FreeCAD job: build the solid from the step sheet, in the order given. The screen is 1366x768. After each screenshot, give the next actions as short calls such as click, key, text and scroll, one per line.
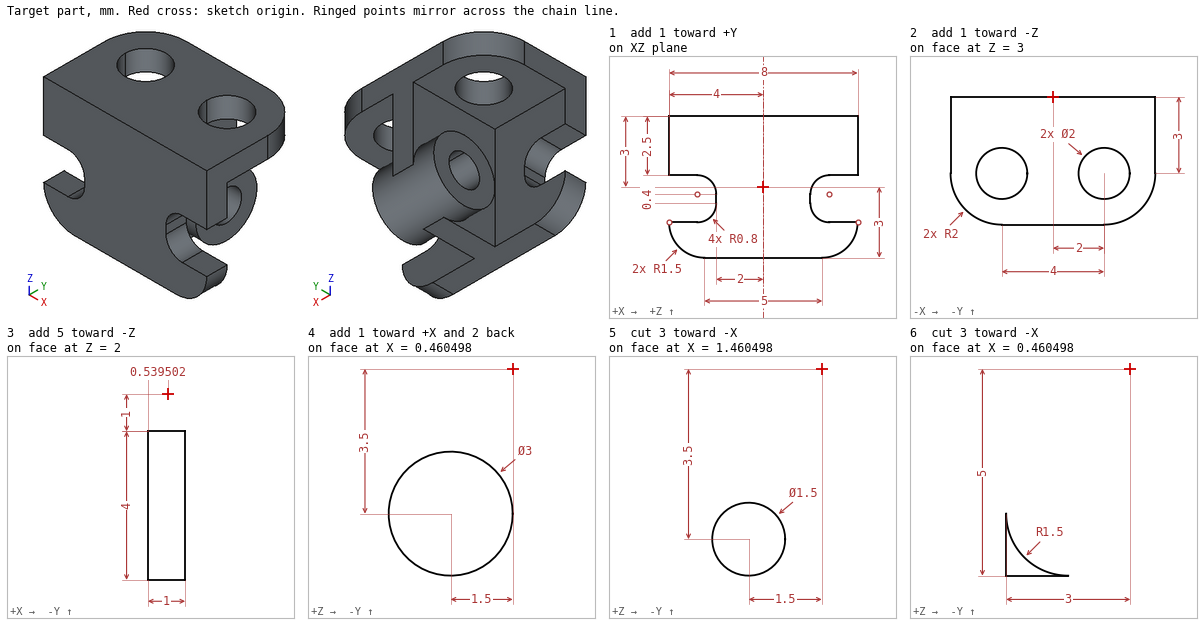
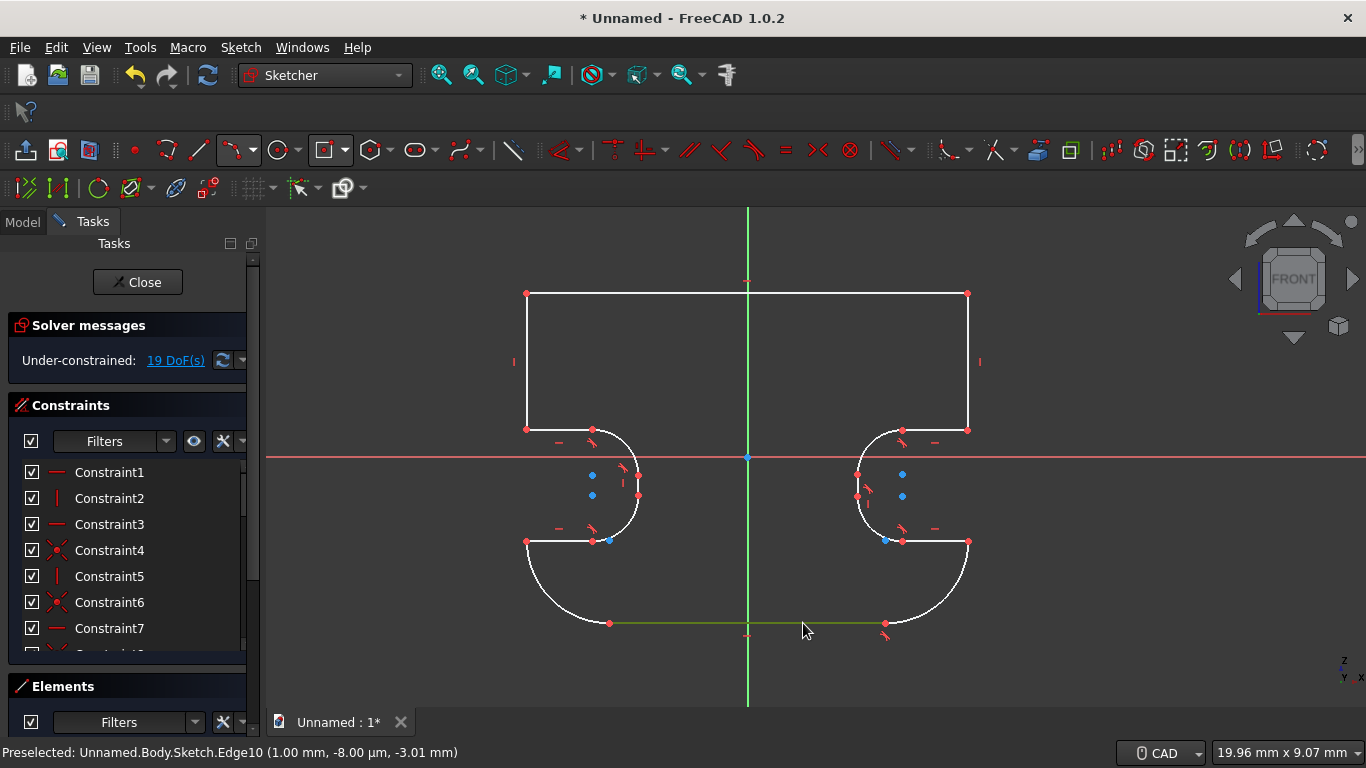
click(536, 579)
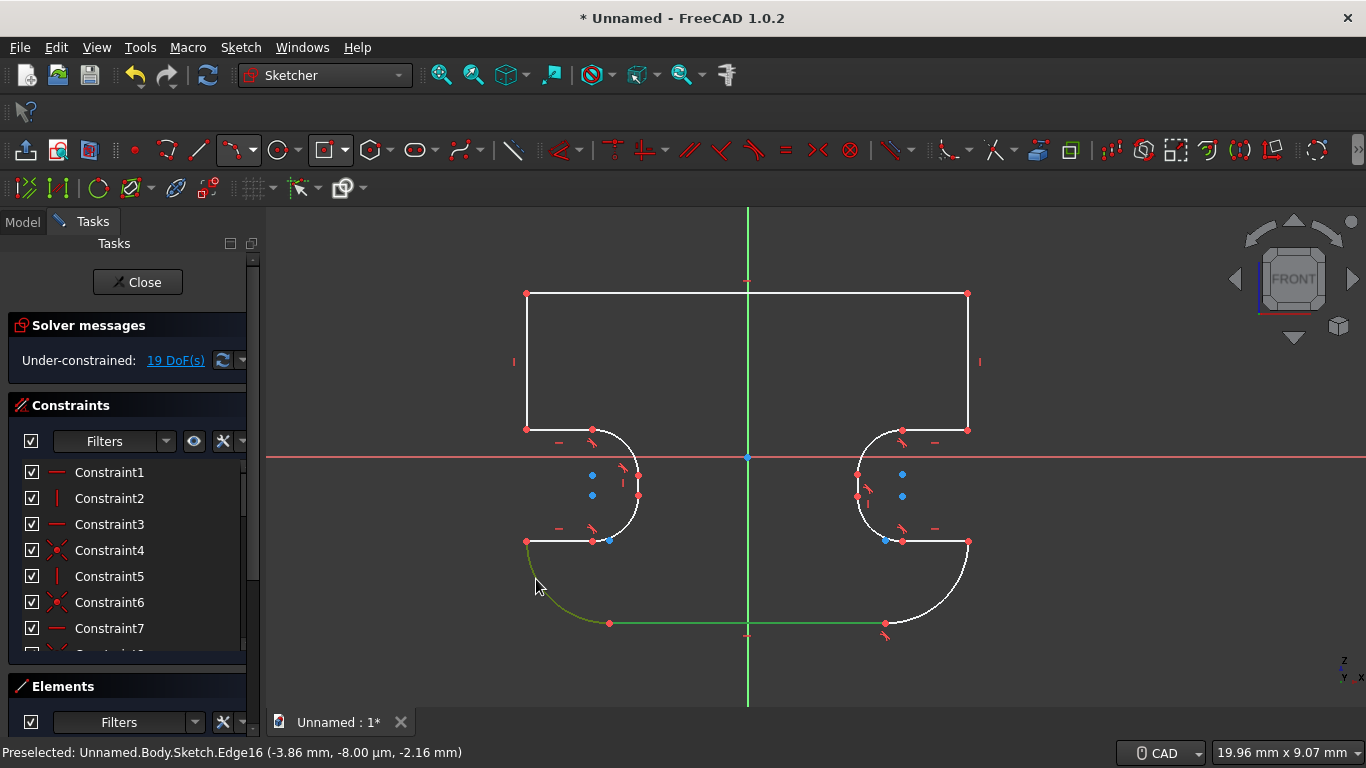
click(754, 150)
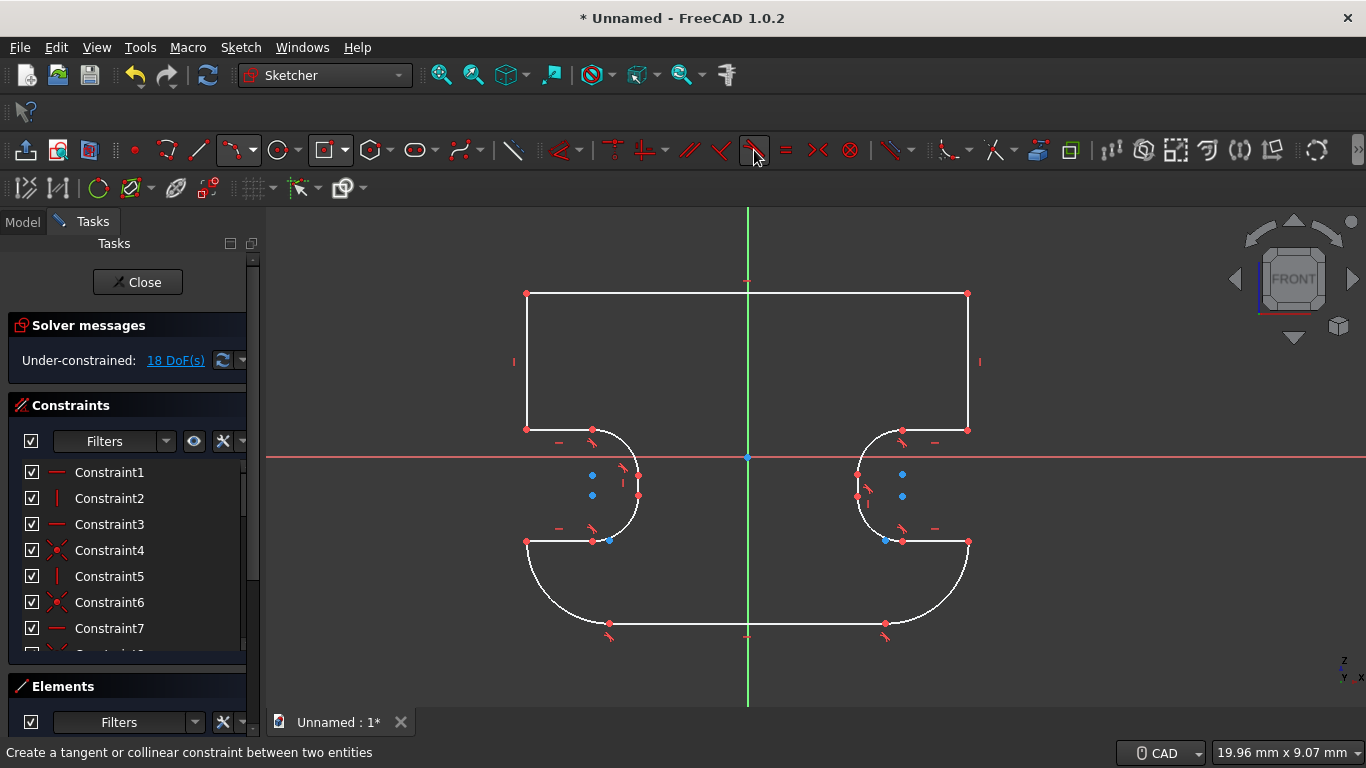
click(633, 516)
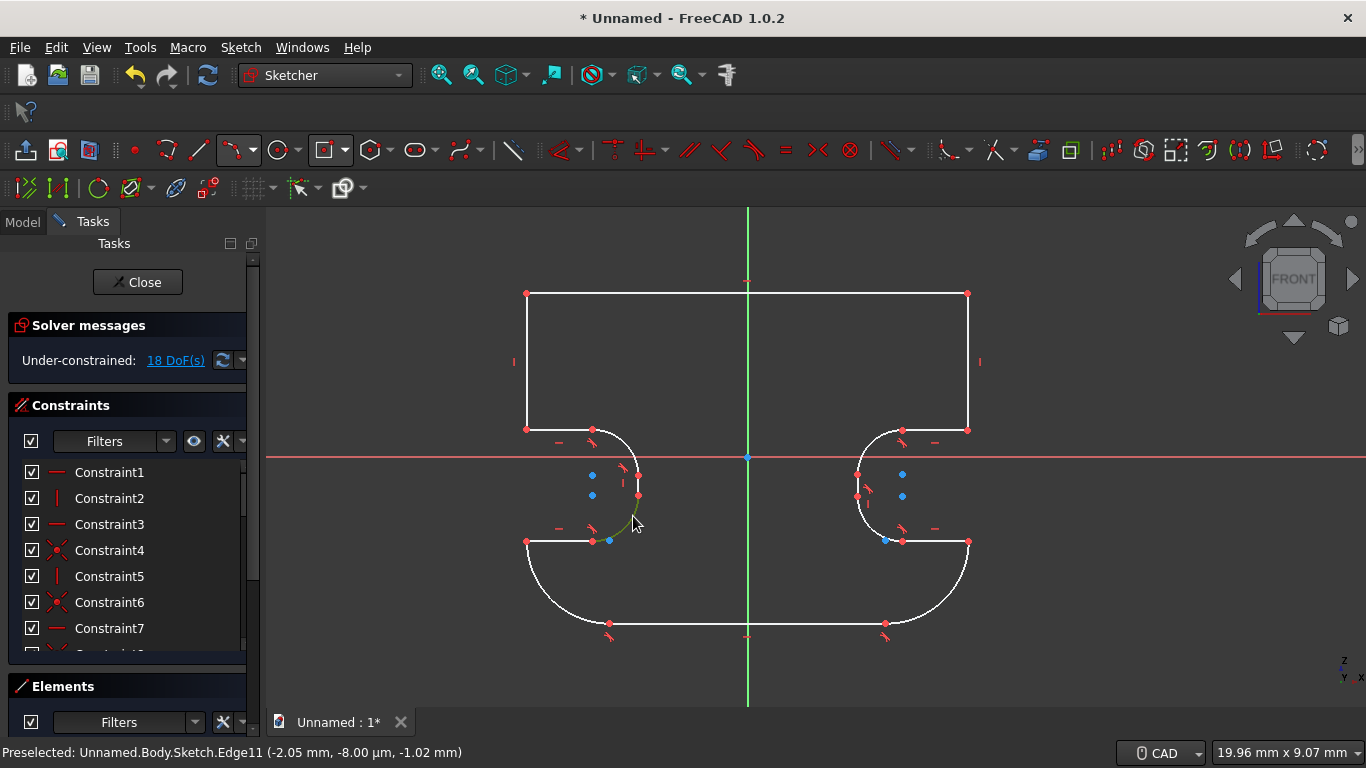
click(633, 455)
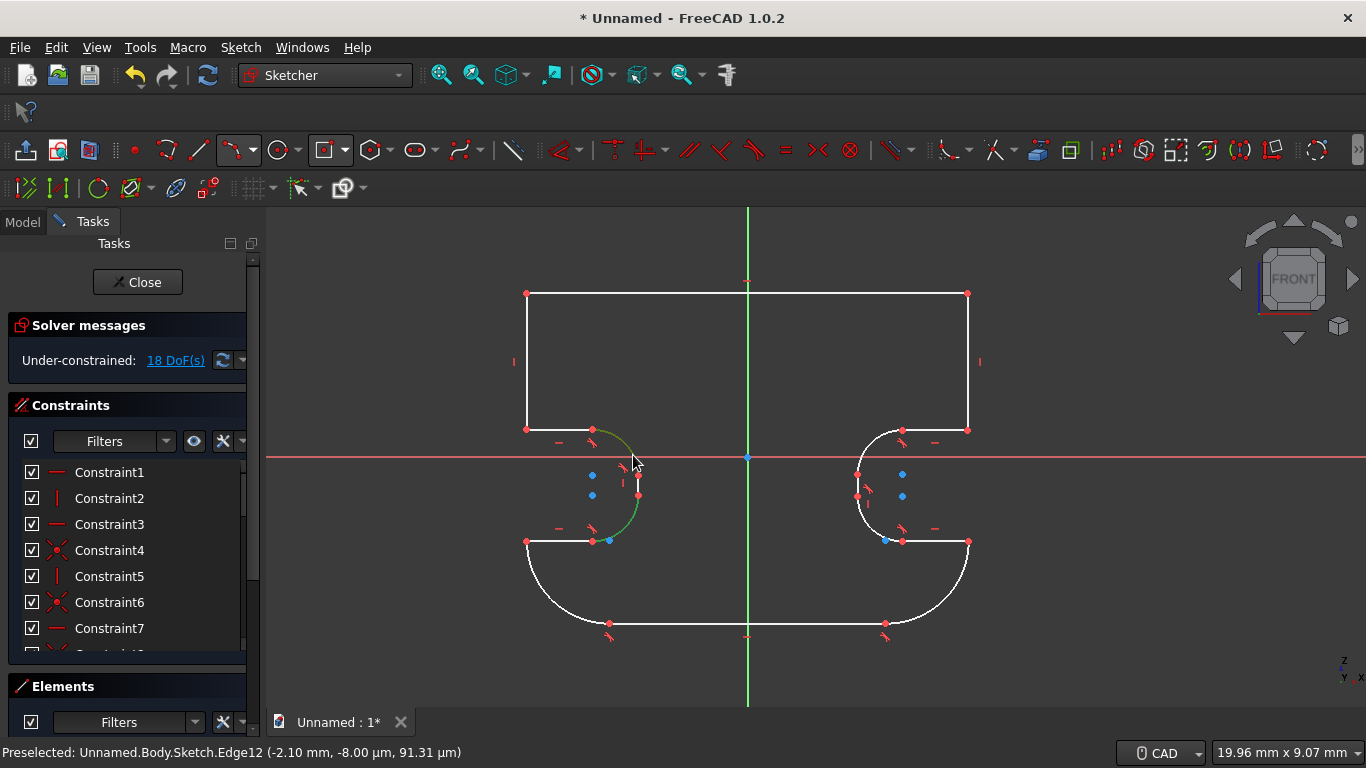
click(882, 435)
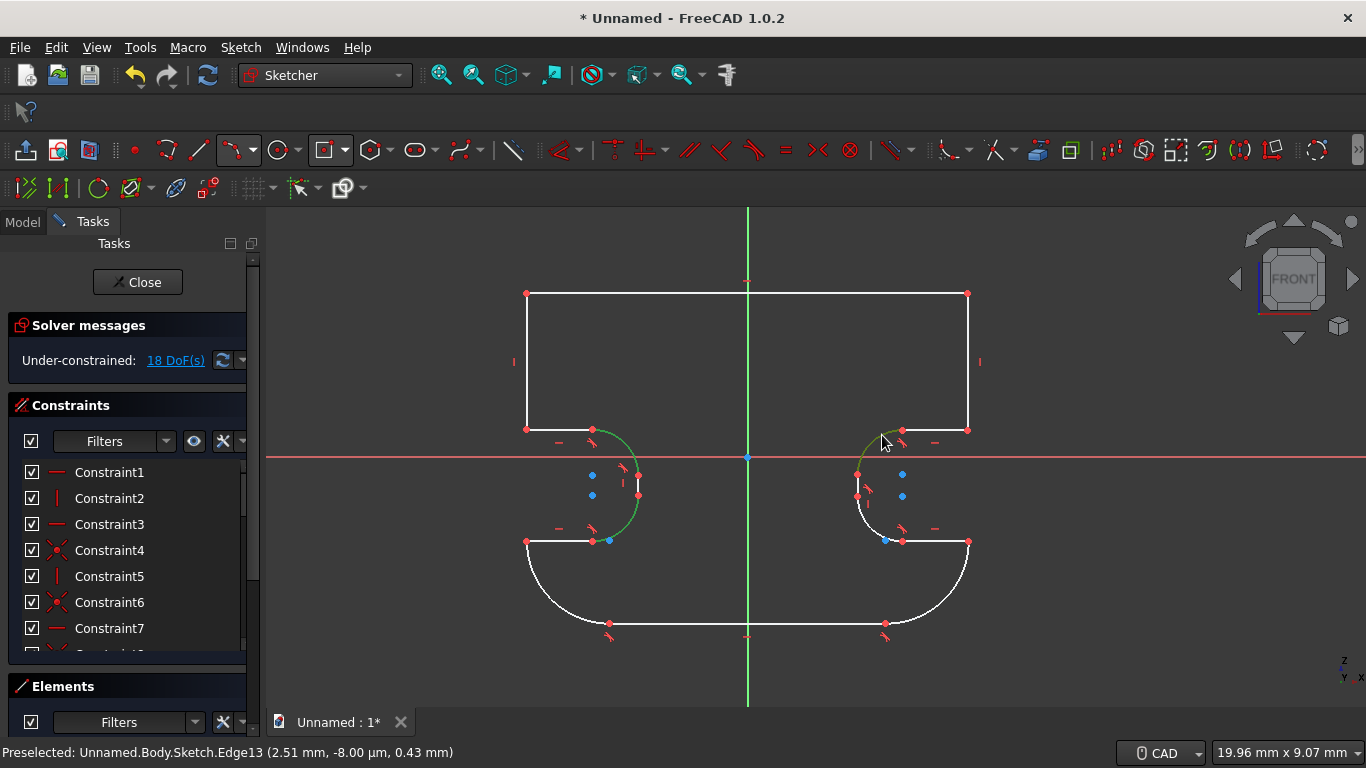
click(863, 517)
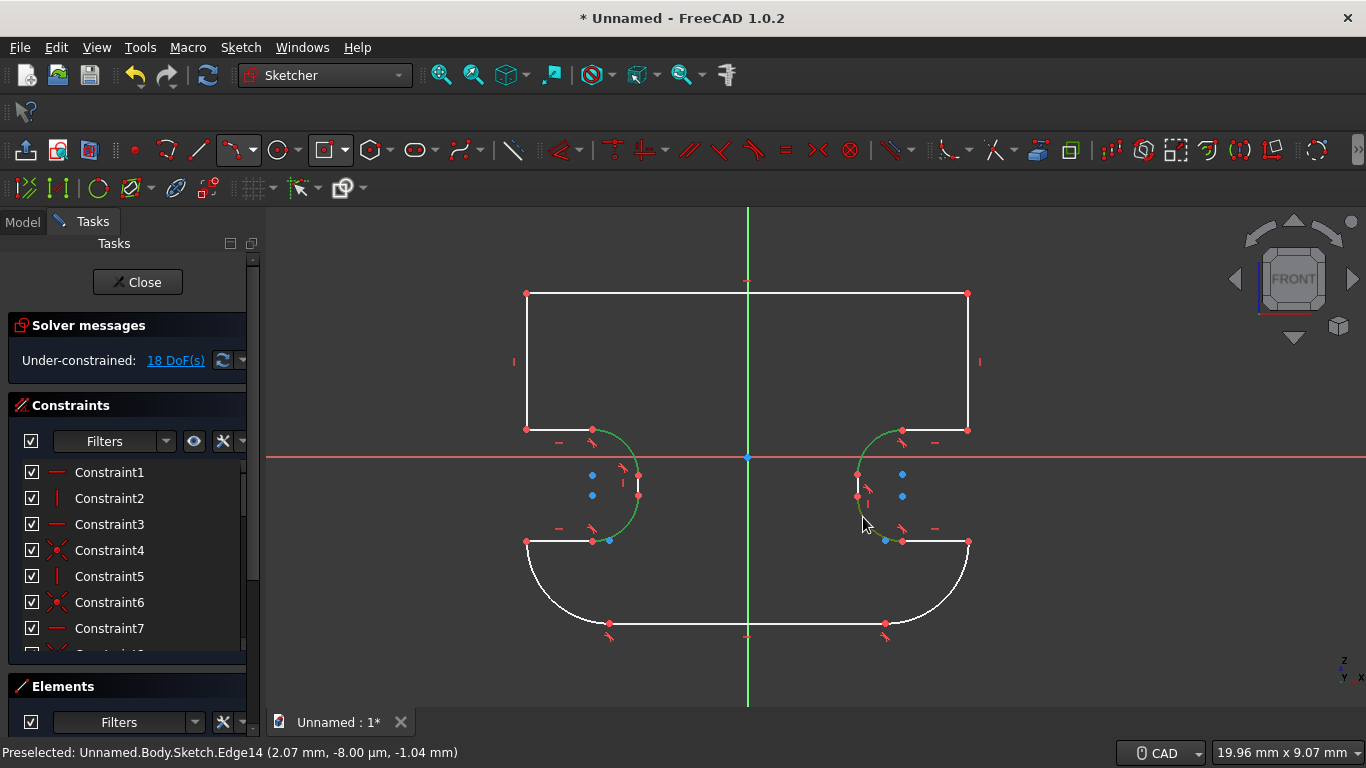
click(786, 150)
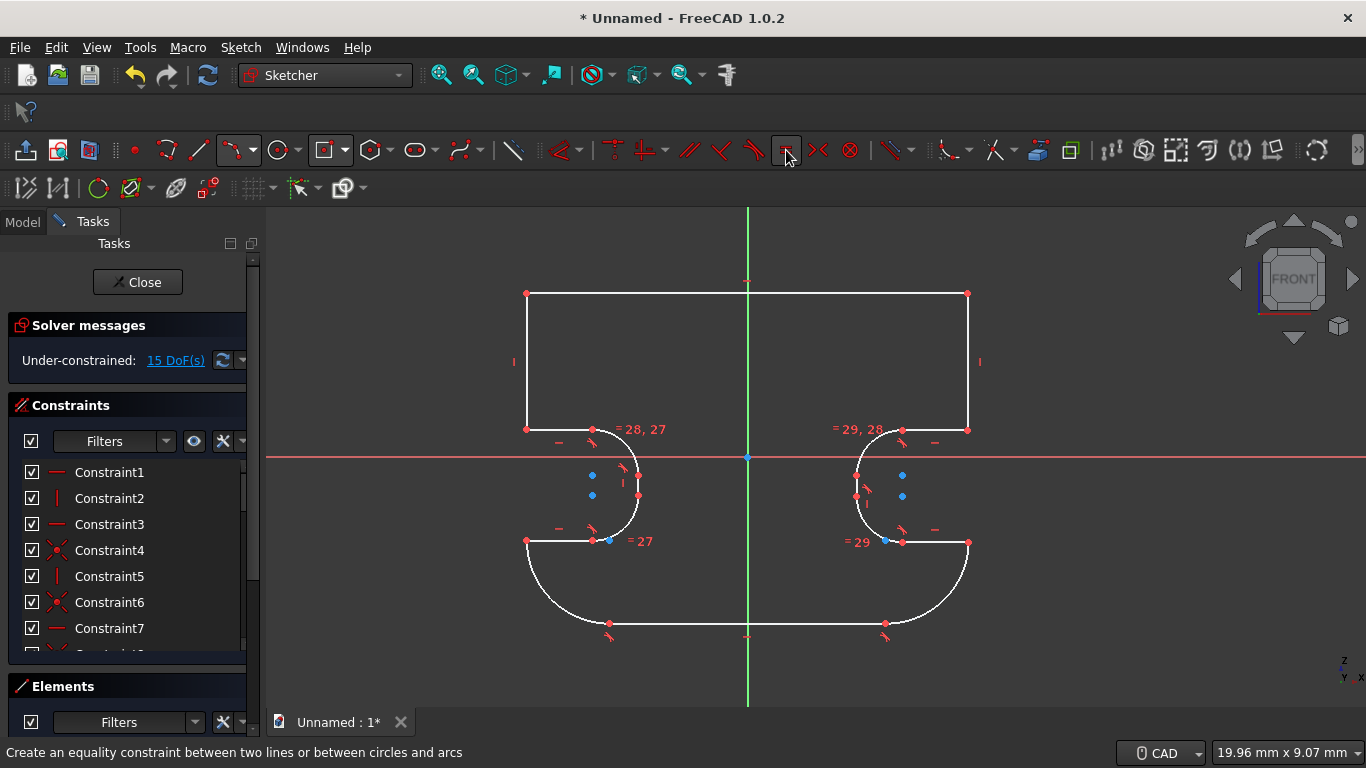
click(923, 615)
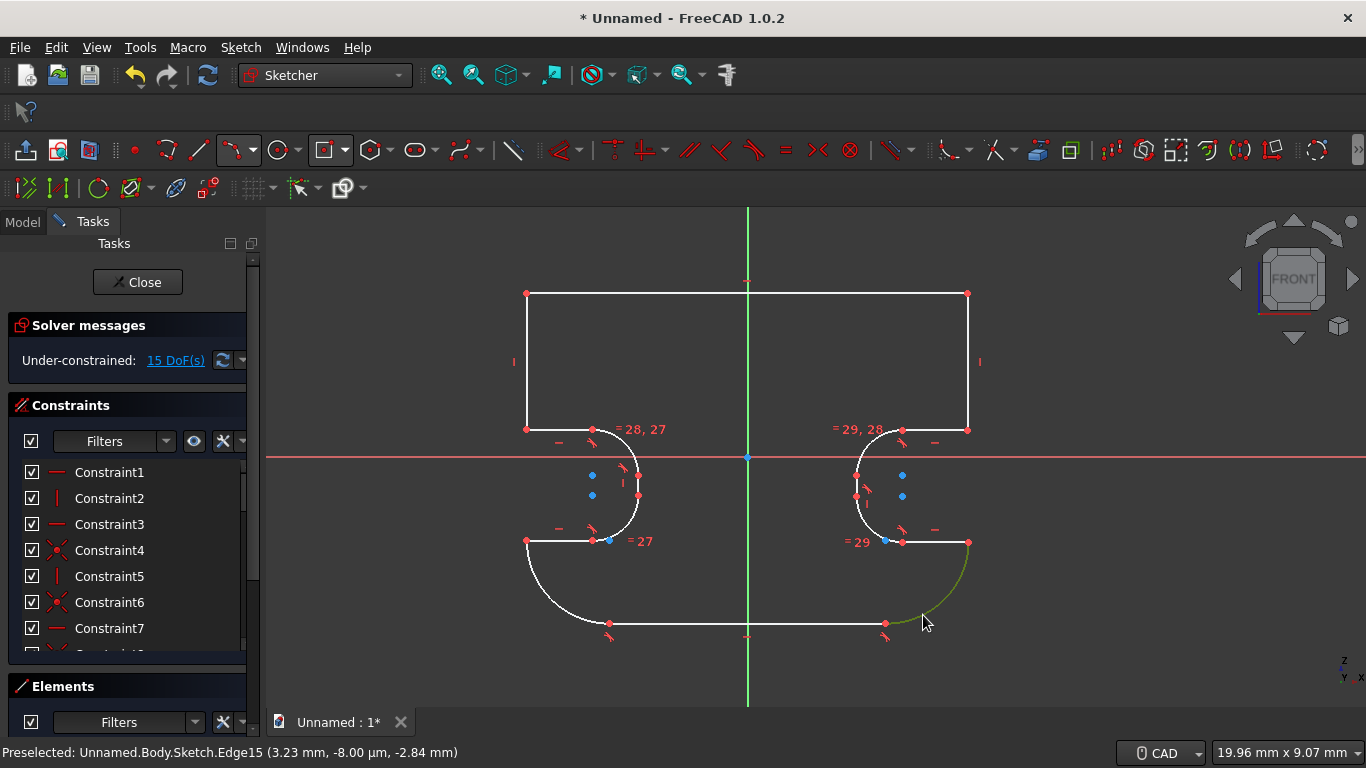
click(536, 578)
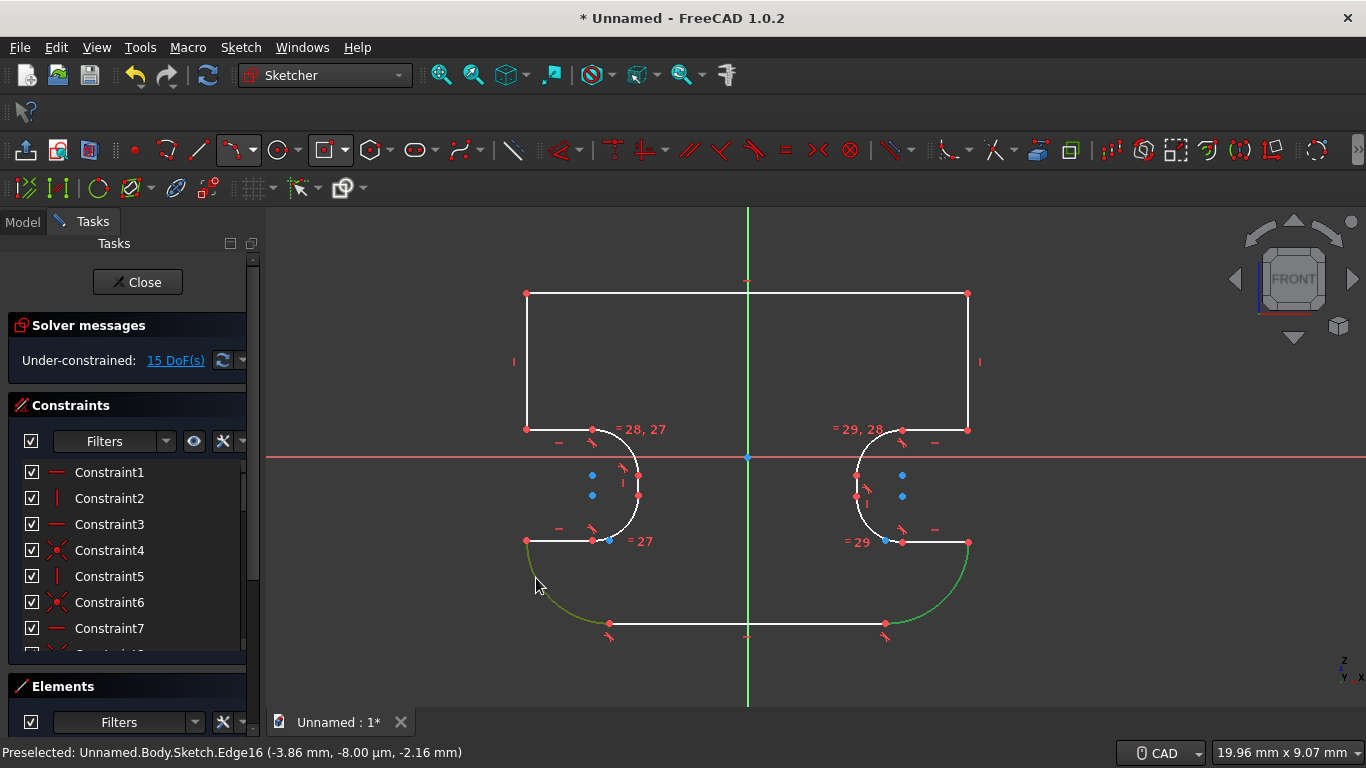
click(786, 150)